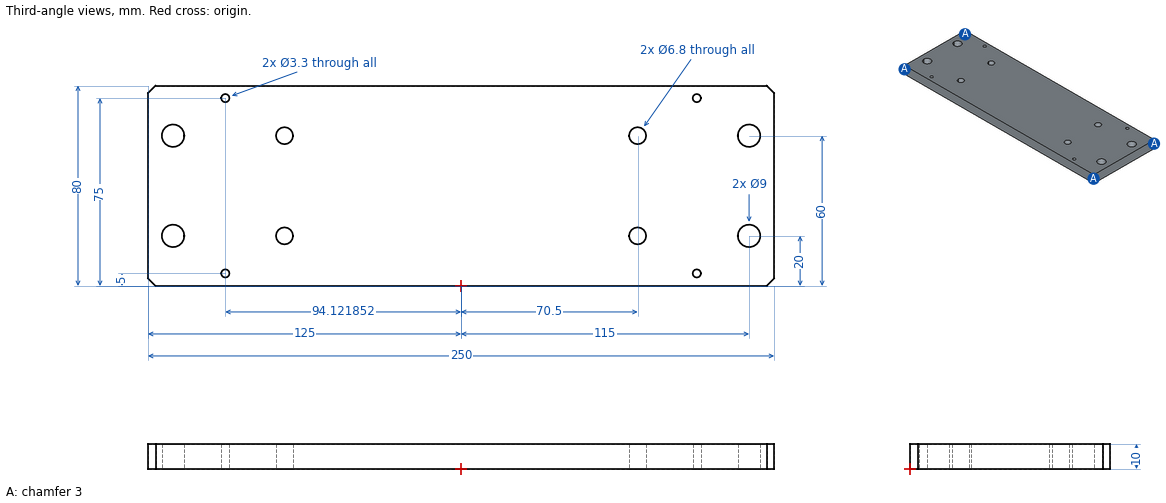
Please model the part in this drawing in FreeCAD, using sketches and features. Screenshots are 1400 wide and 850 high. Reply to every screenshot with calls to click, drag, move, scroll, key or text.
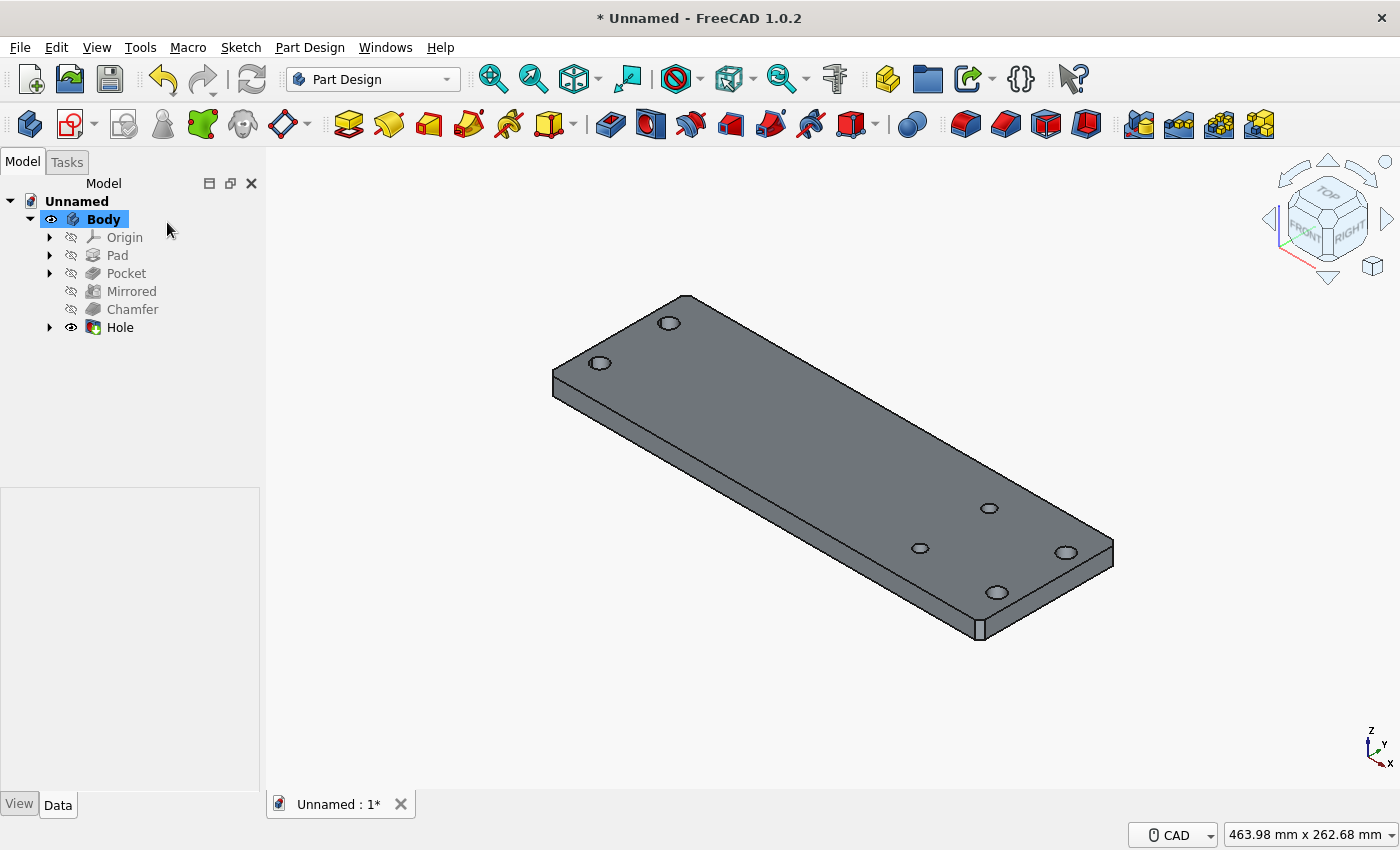
click(116, 327)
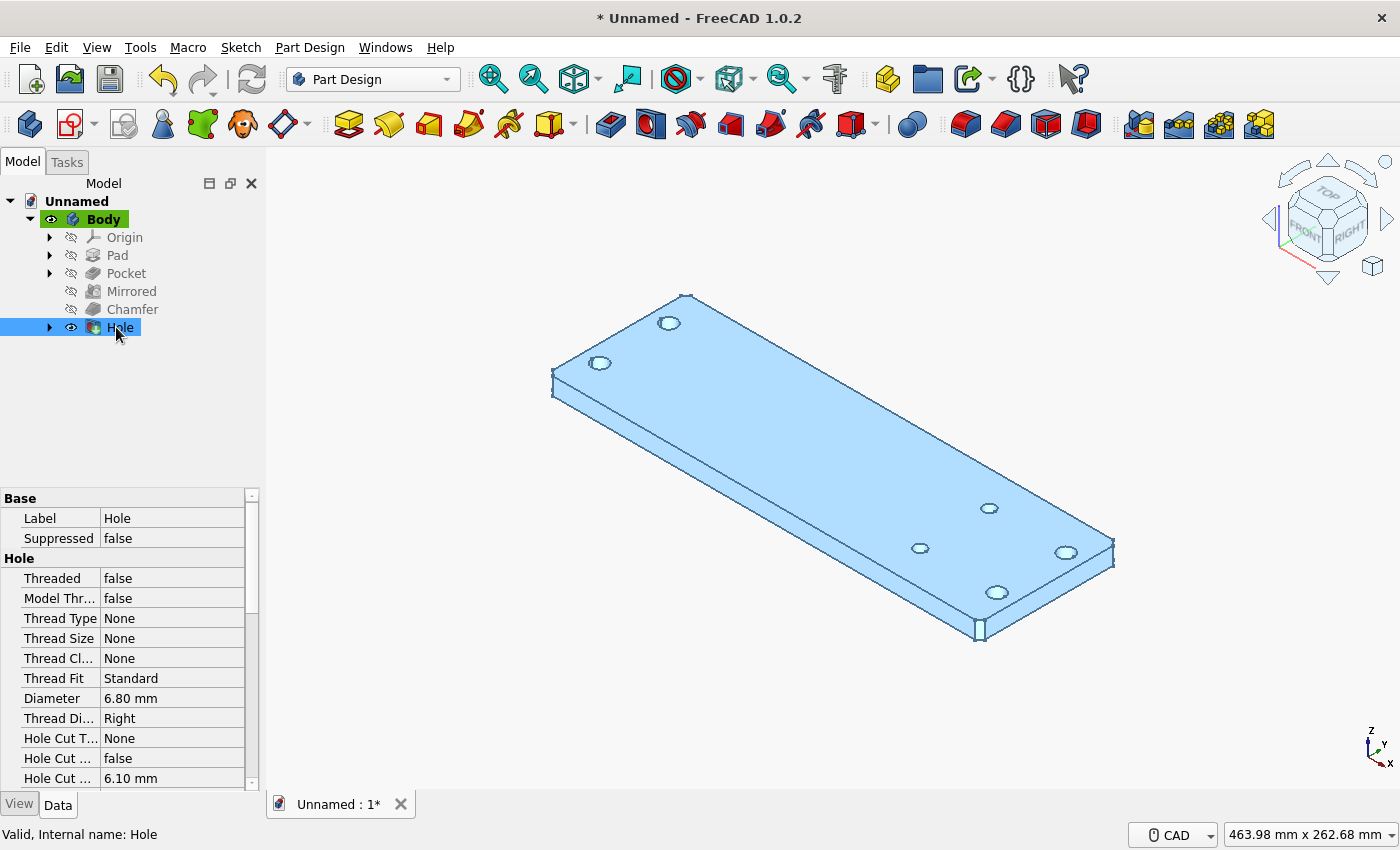
click(1140, 124)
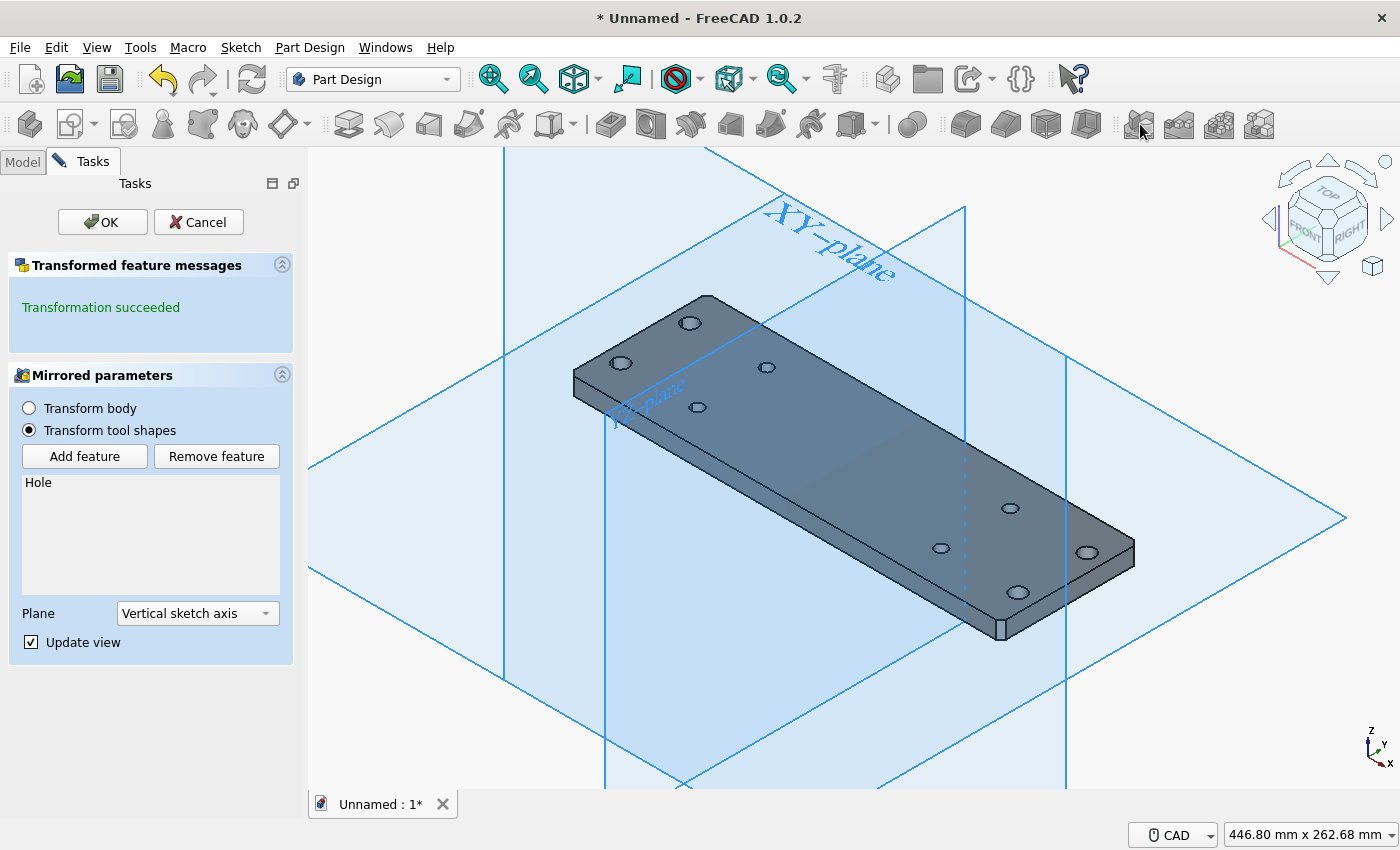
click(198, 614)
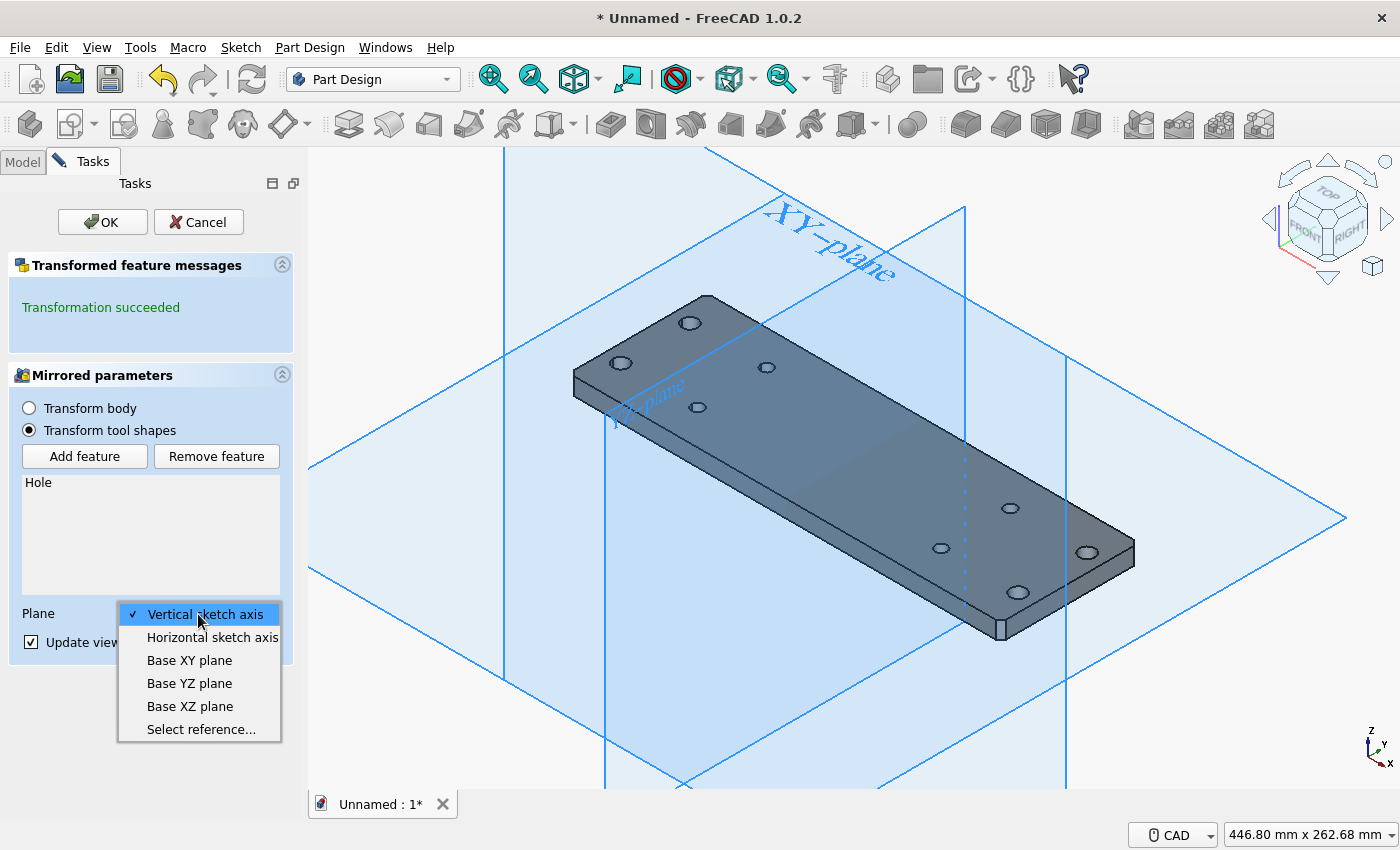
click(198, 684)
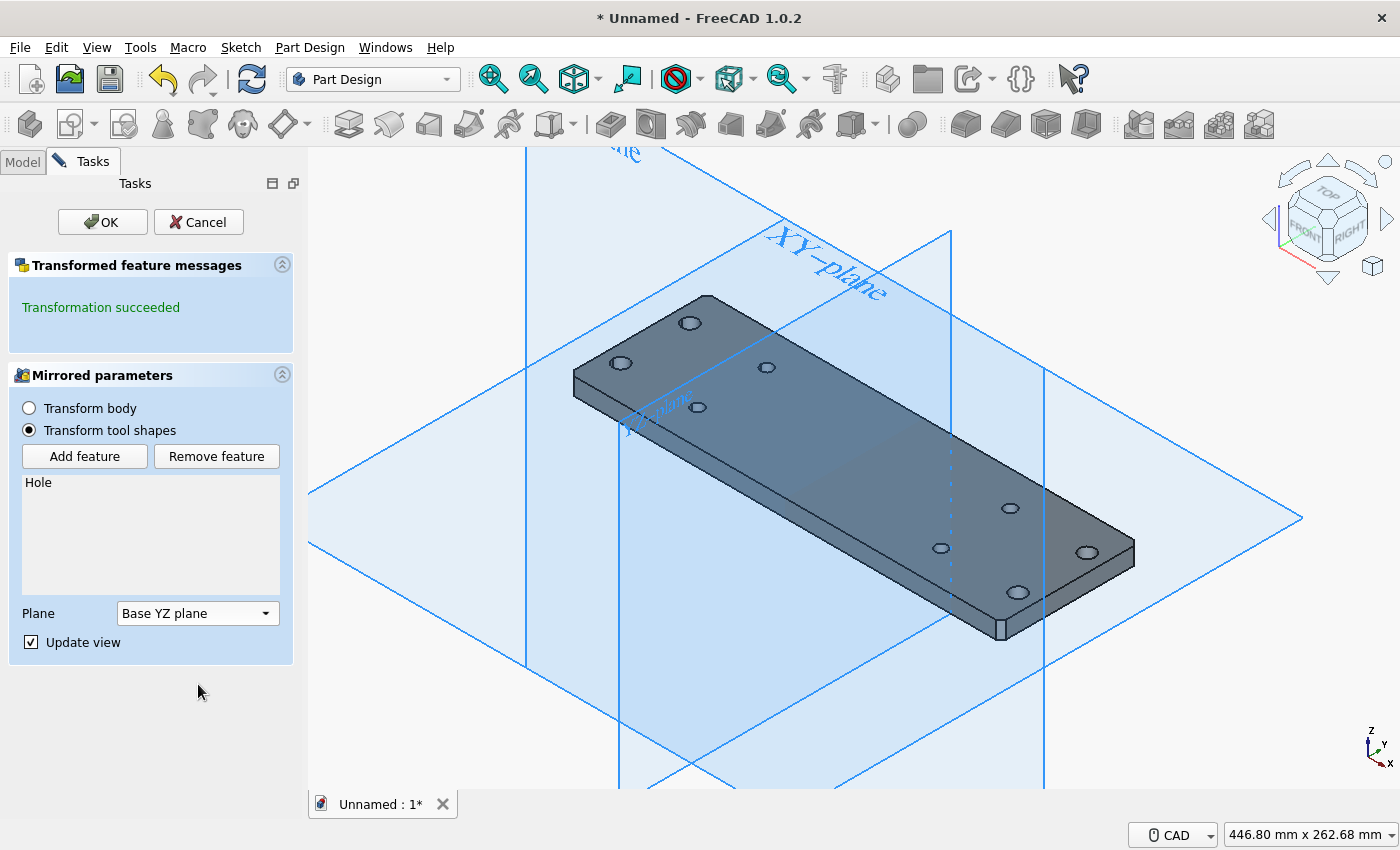
click(103, 222)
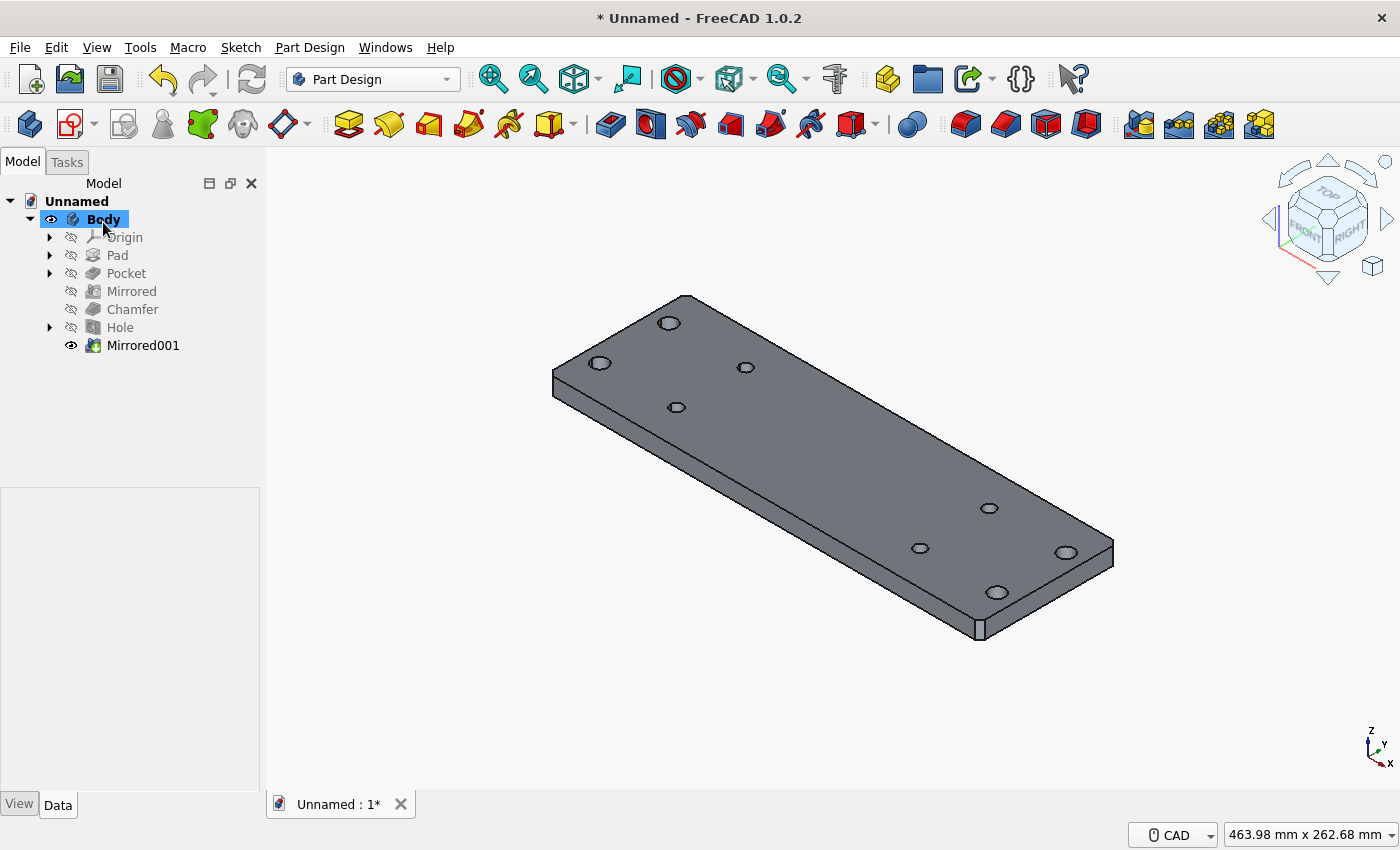
click(833, 457)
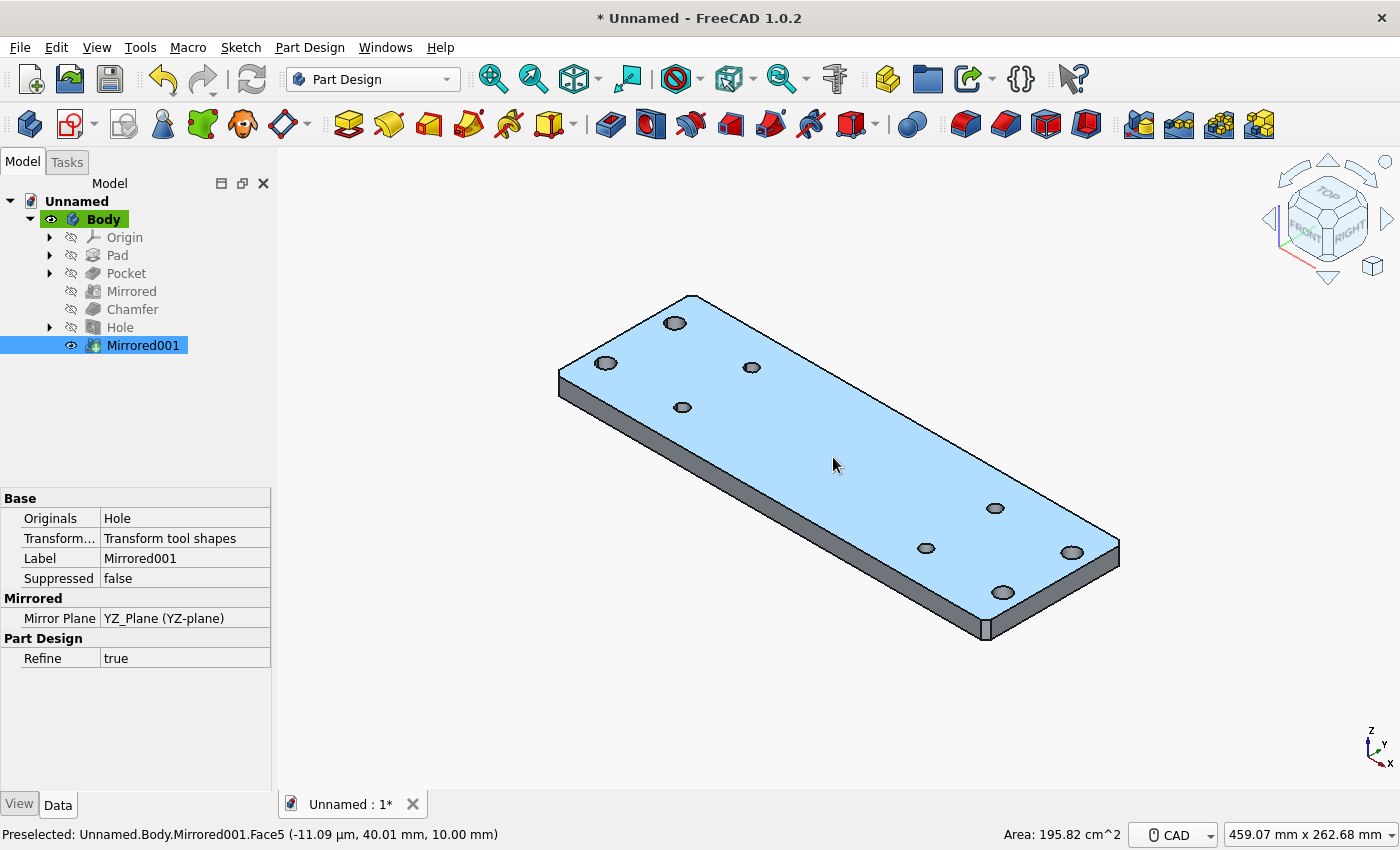
click(70, 124)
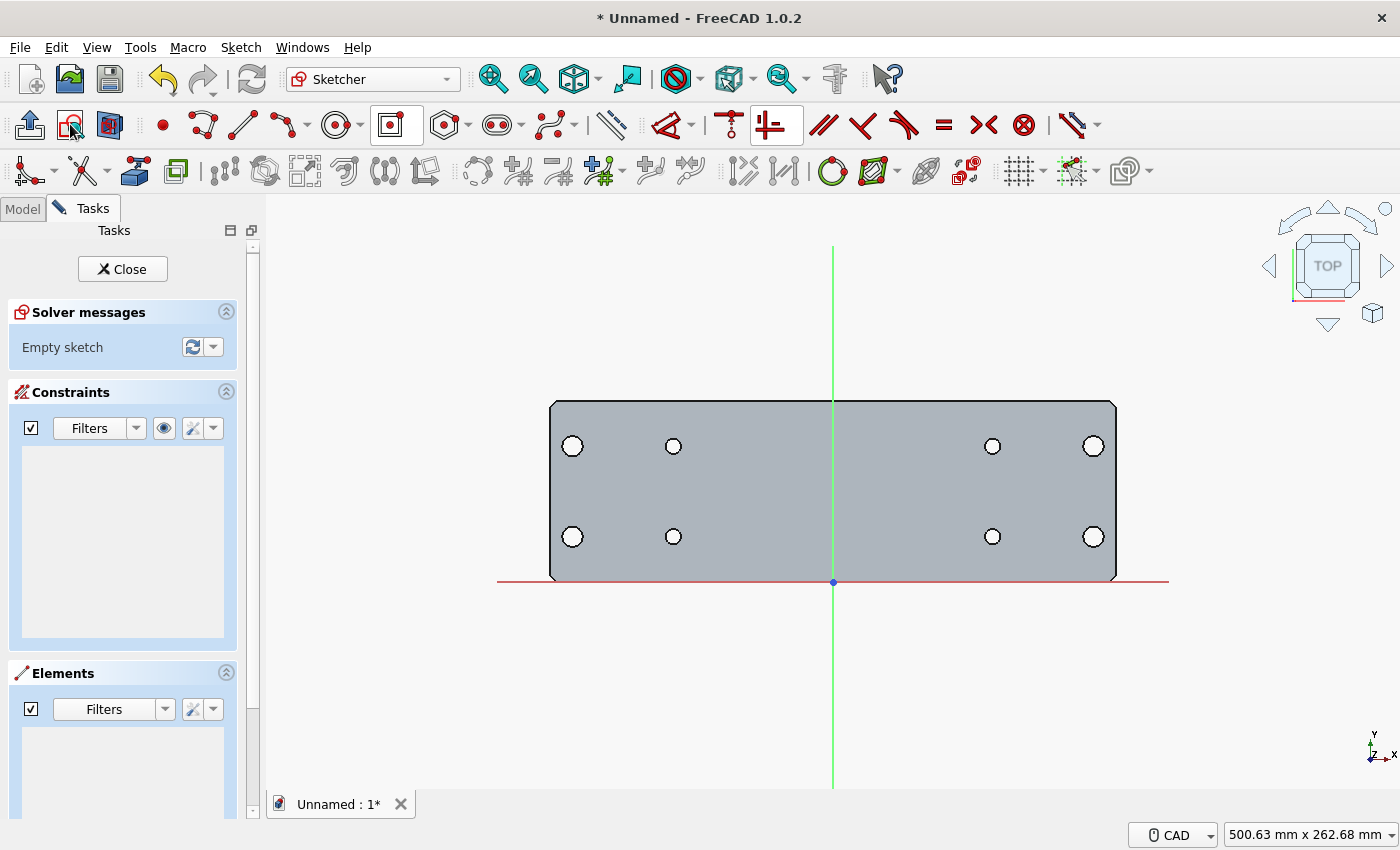
scroll(692, 498, up, 4)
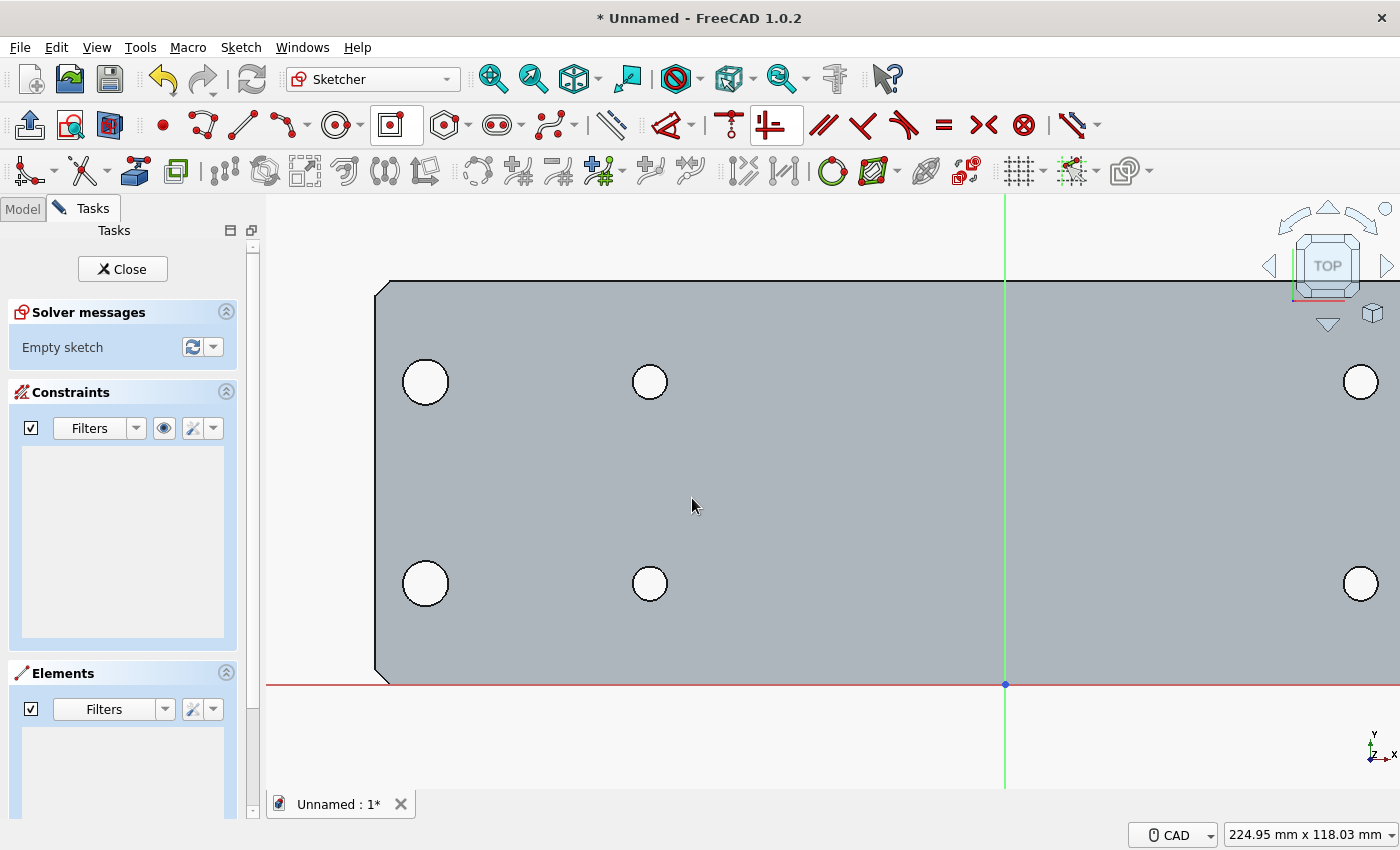
click(336, 126)